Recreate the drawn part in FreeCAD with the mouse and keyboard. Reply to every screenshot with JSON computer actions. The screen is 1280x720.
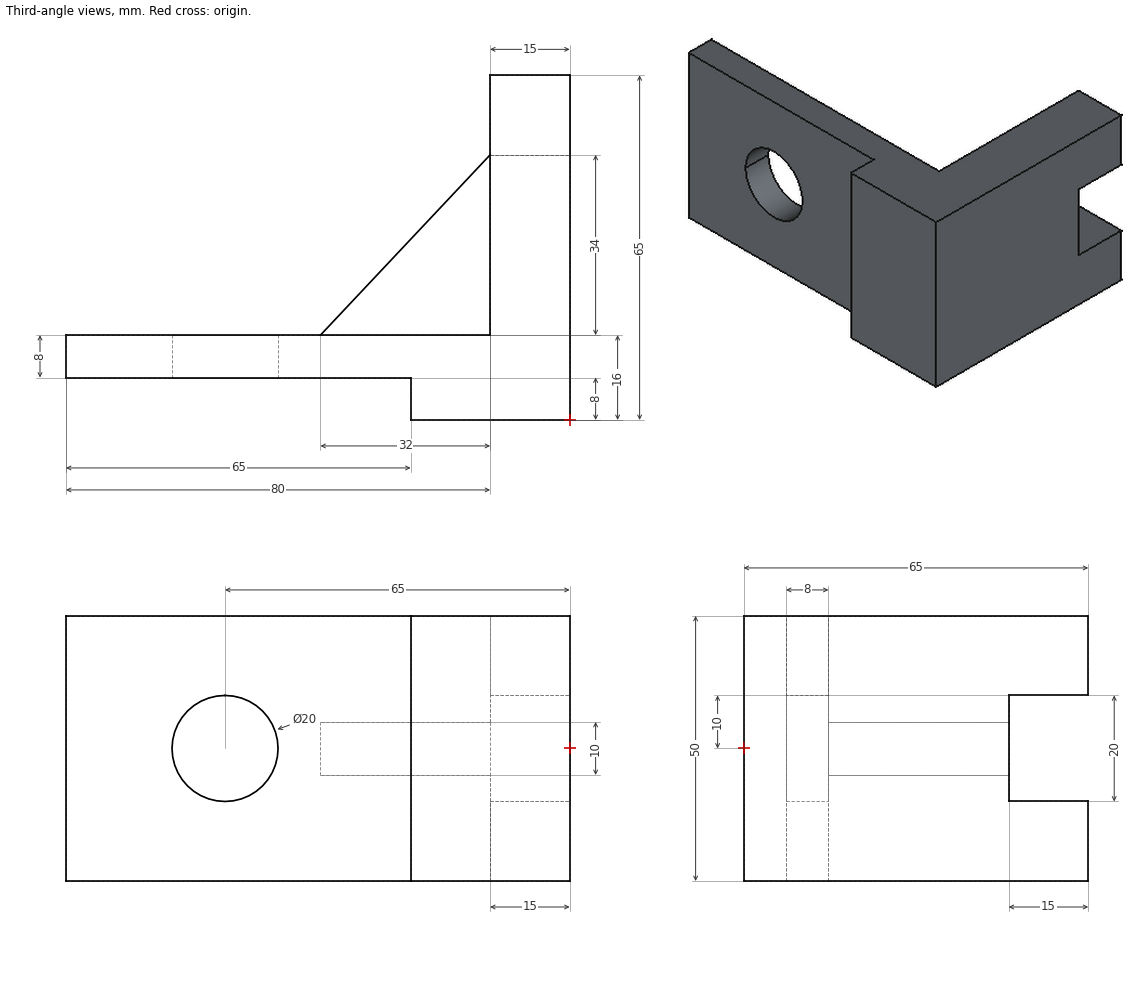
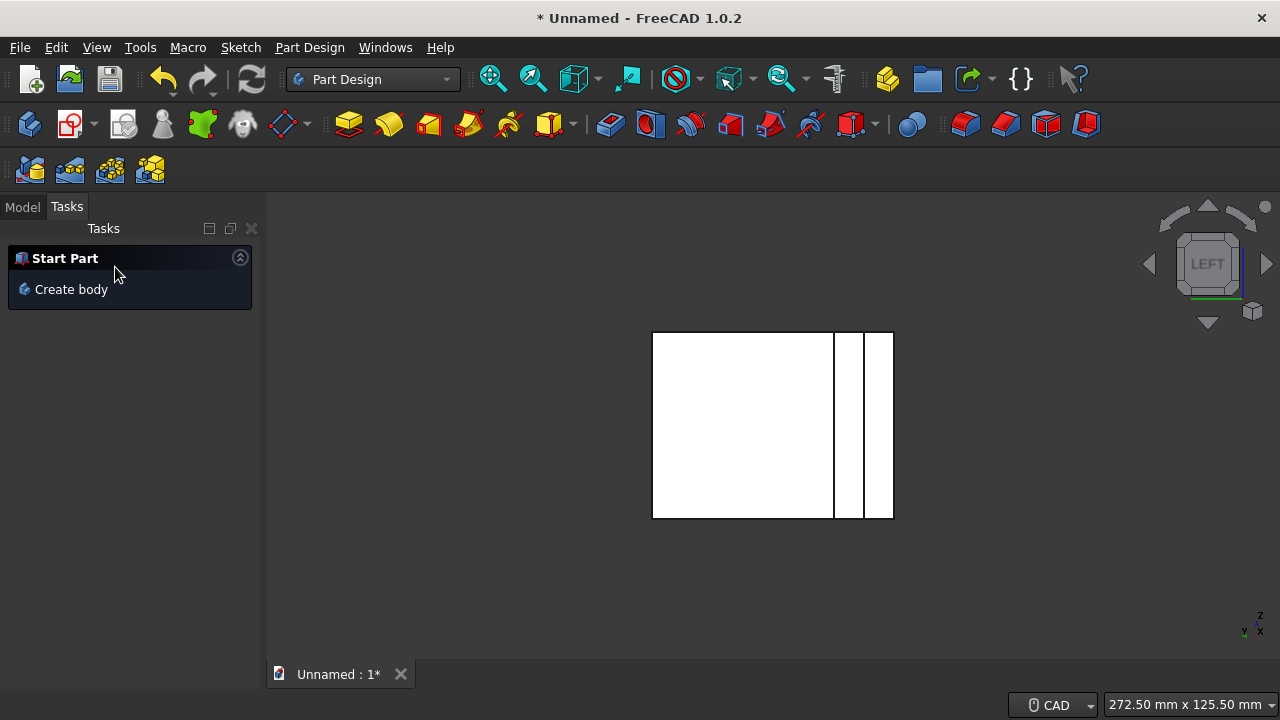
{"action": "left_click", "coordinate": [743, 424]}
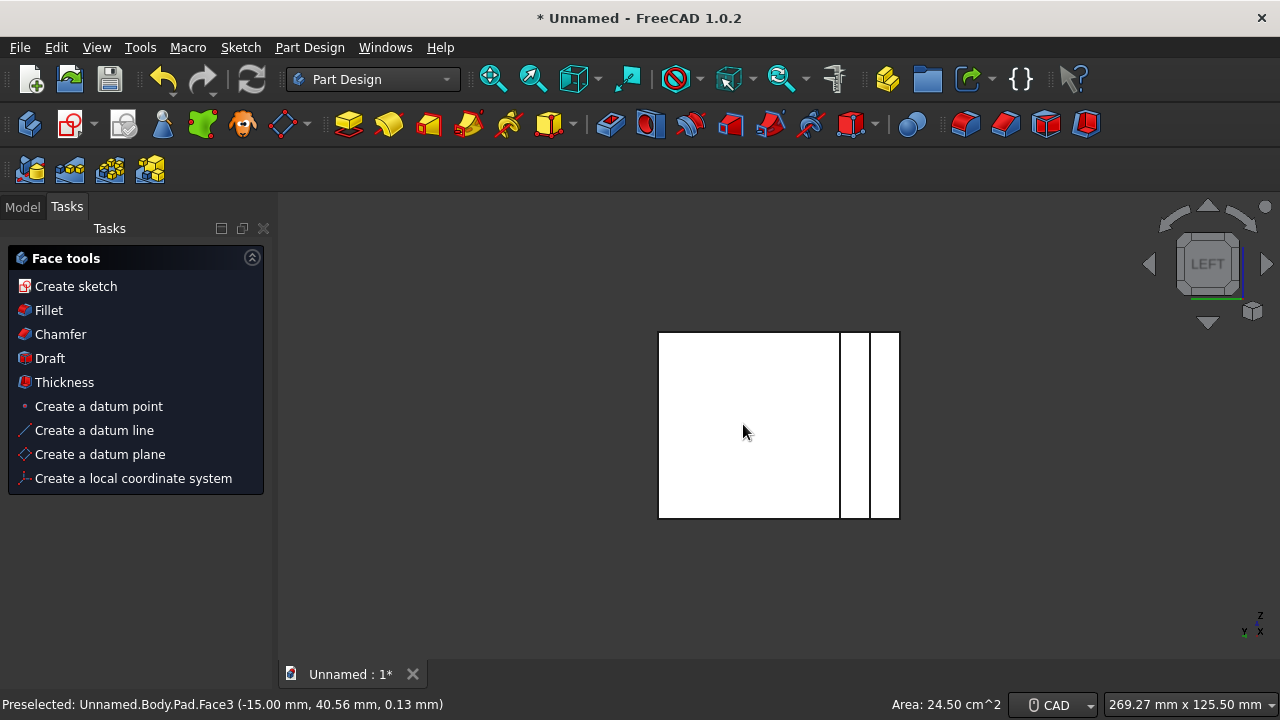
{"action": "left_click", "coordinate": [70, 124]}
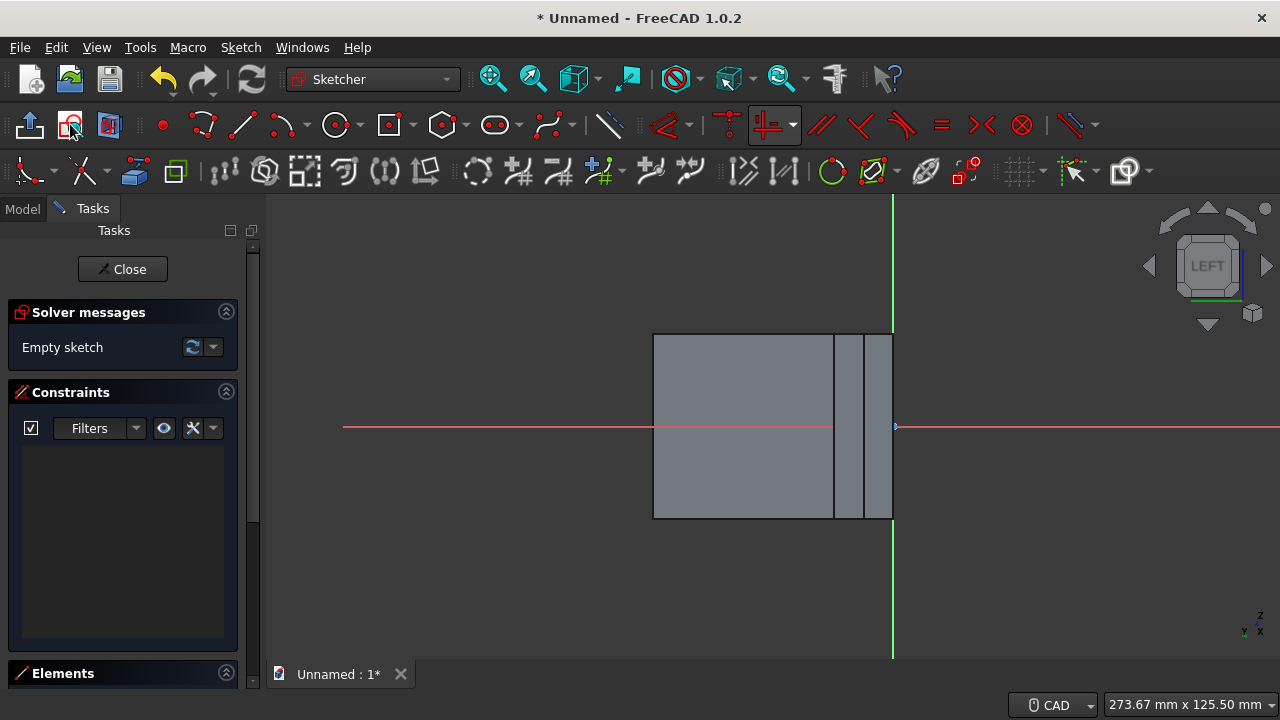
{"action": "scroll", "coordinate": [672, 426], "scroll_direction": "up", "scroll_amount": 7}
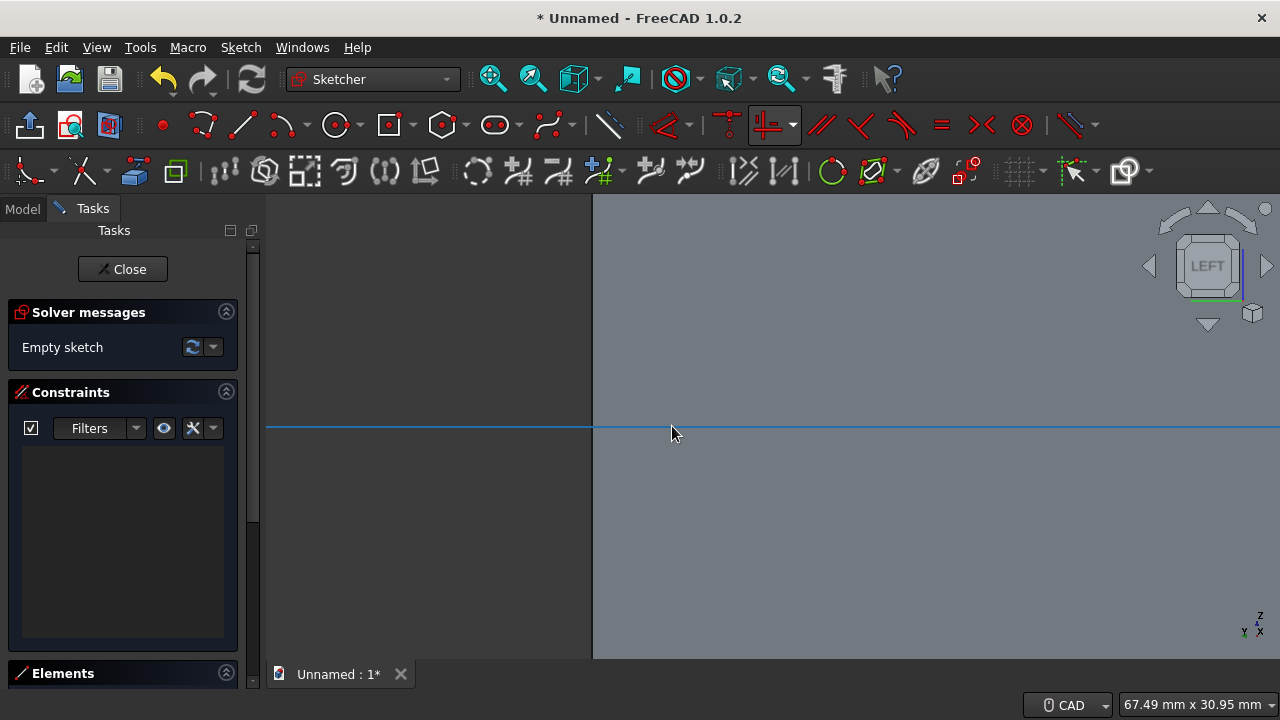
{"action": "left_click", "coordinate": [416, 126]}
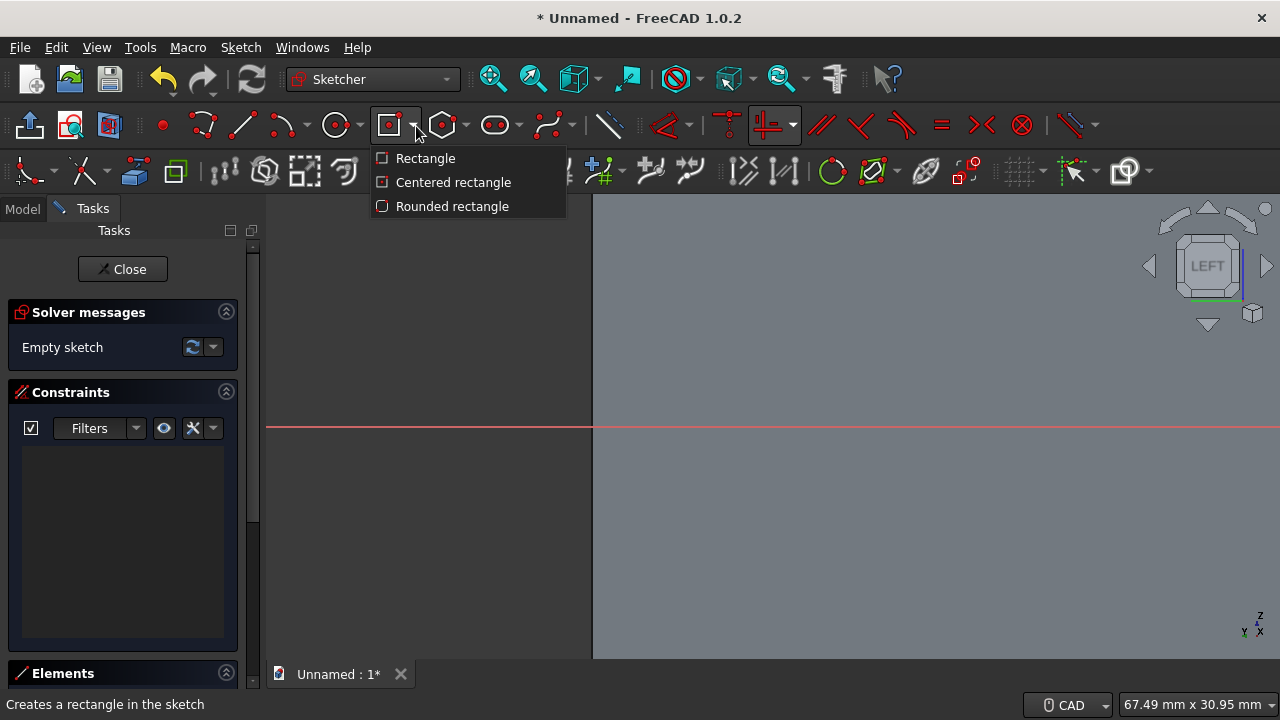
{"action": "left_click", "coordinate": [468, 158]}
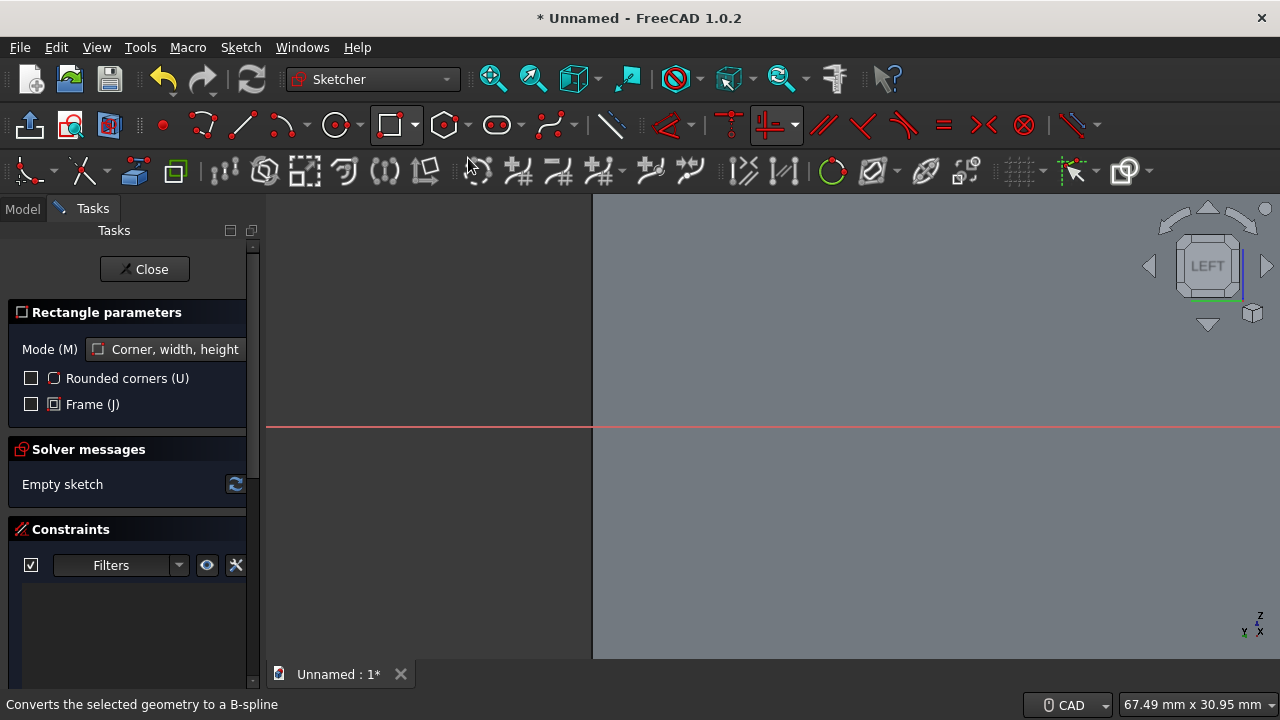
{"action": "left_click", "coordinate": [592, 276]}
{"action": "mouse_move", "coordinate": [817, 577]}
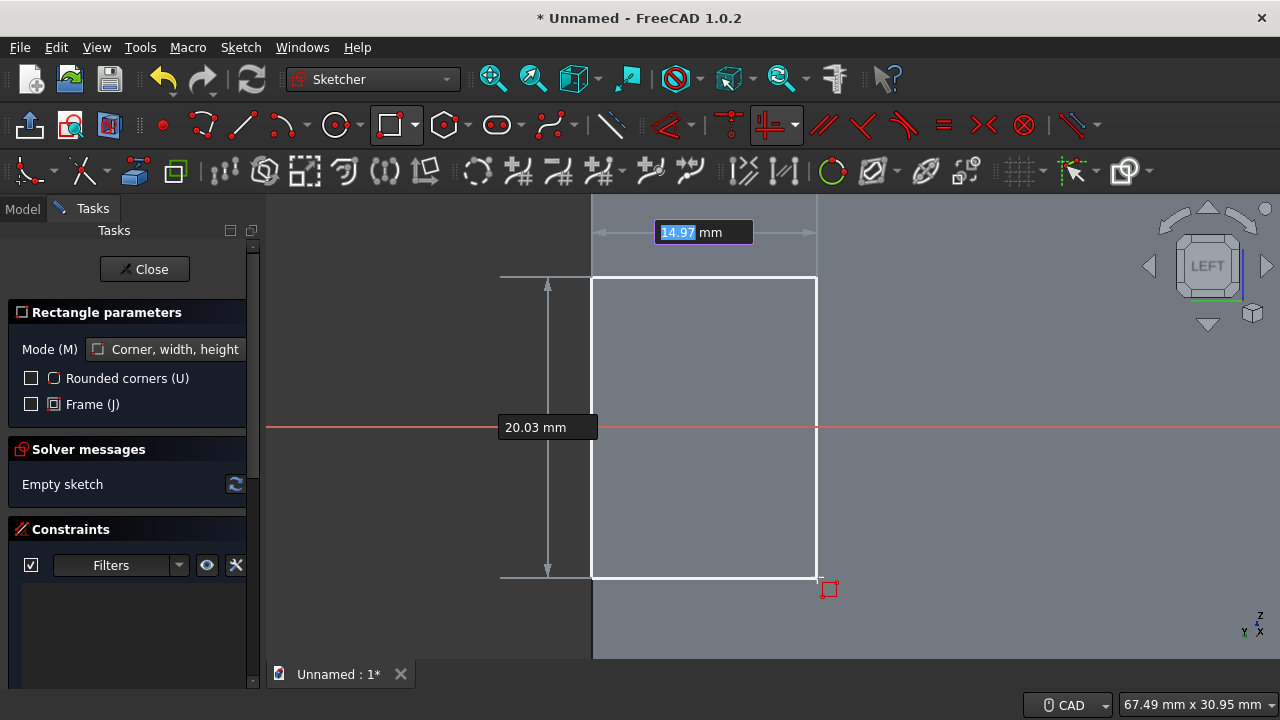
{"action": "type", "text": "15"}
{"action": "key", "text": "Tab"}
{"action": "type", "text": "20"}
{"action": "key", "text": "Return"}
{"action": "key", "text": "Escape"}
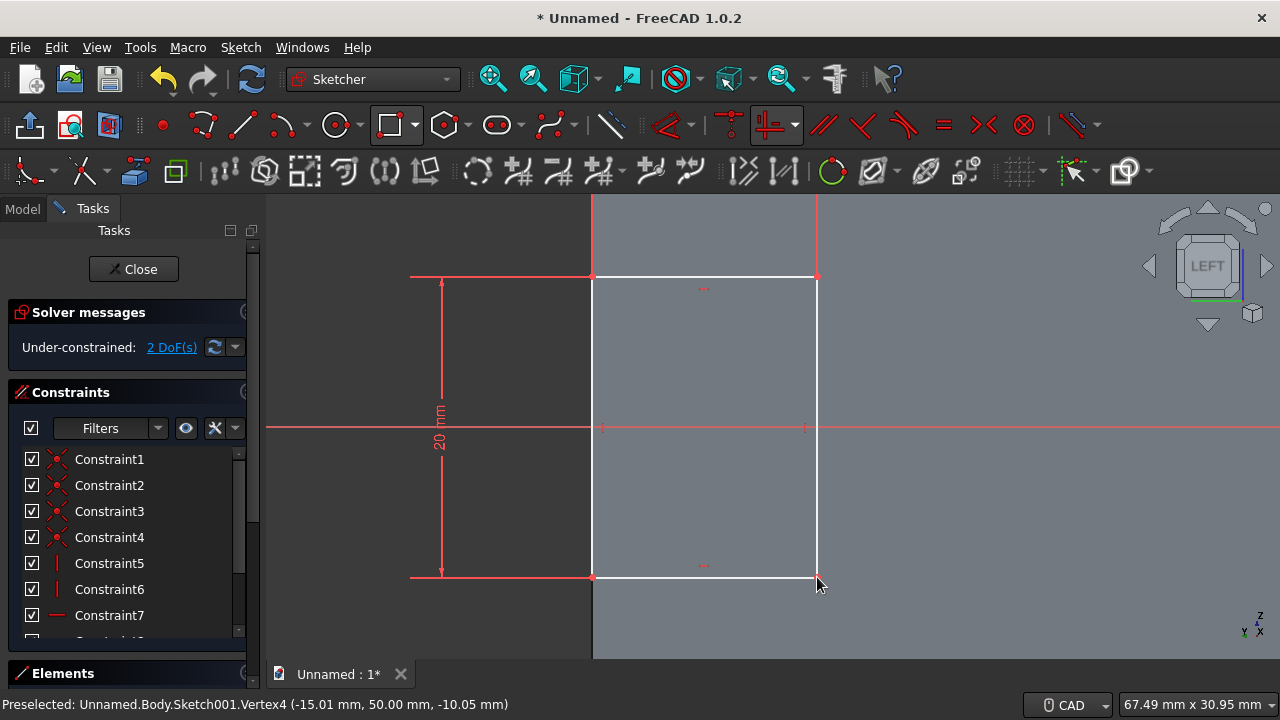
{"action": "key", "text": "d"}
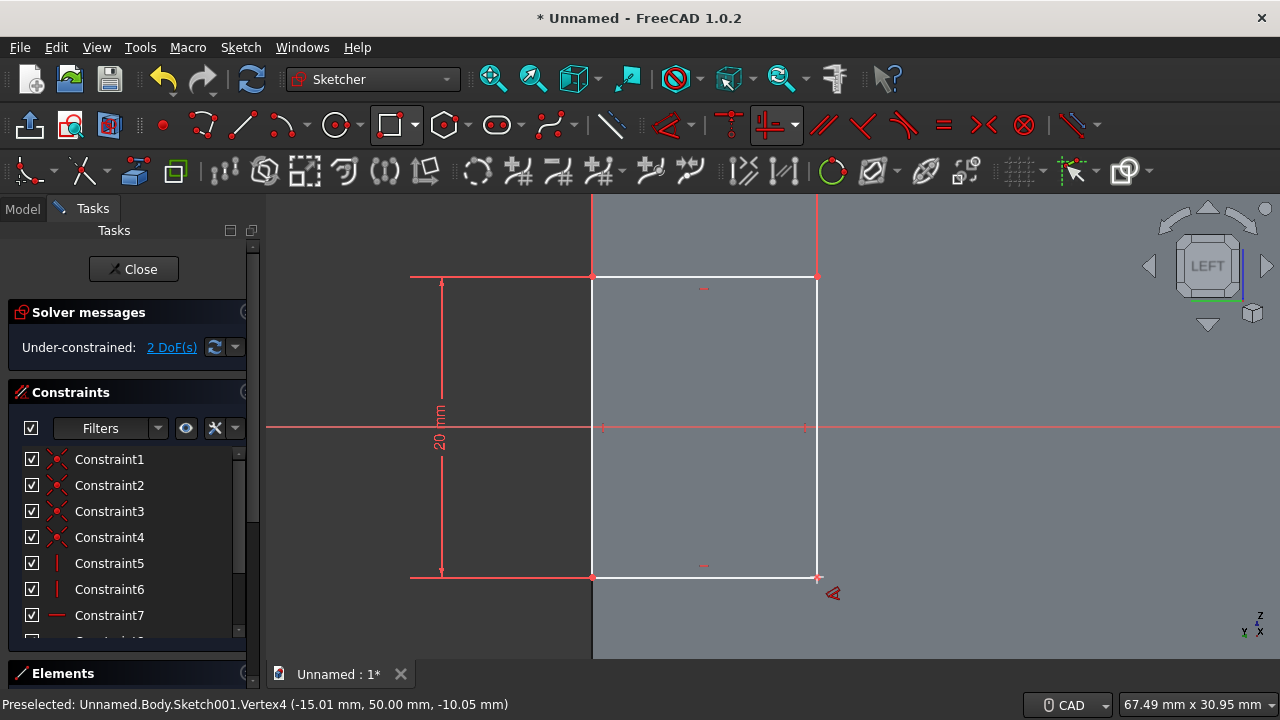
{"action": "left_click", "coordinate": [592, 277]}
{"action": "left_click", "coordinate": [853, 243]}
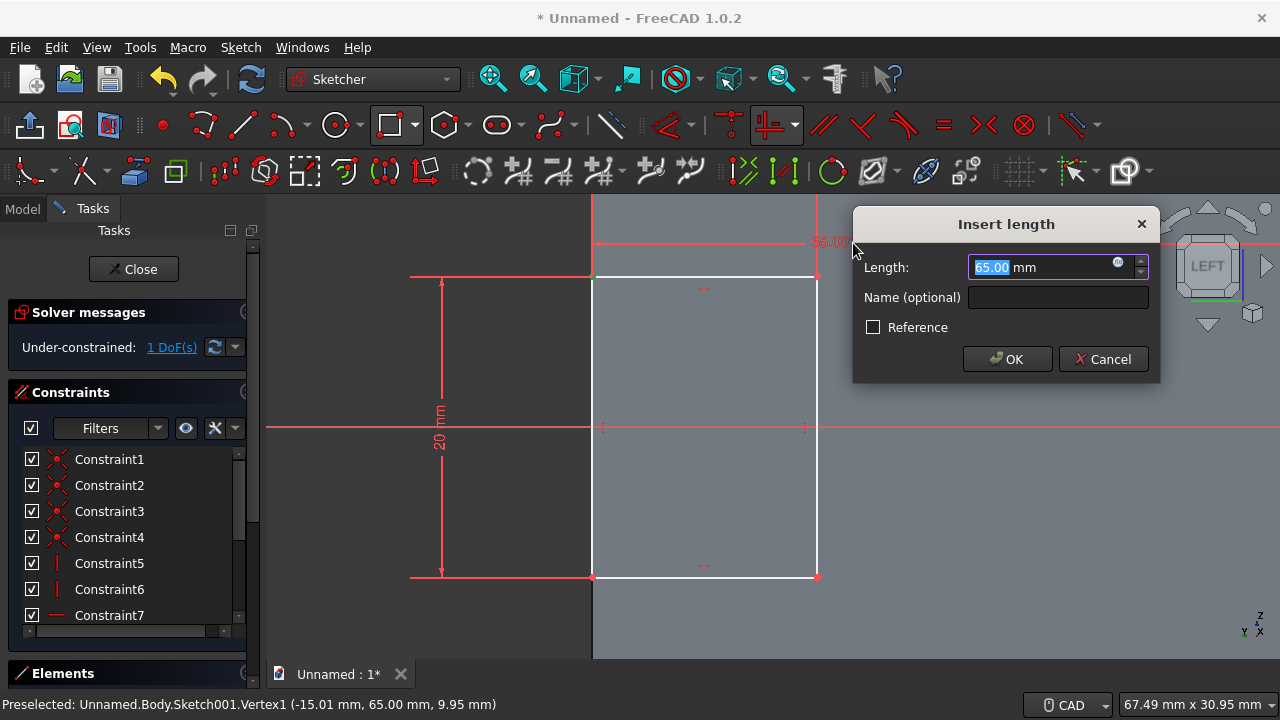
{"action": "type", "text": "65"}
{"action": "key", "text": "Return"}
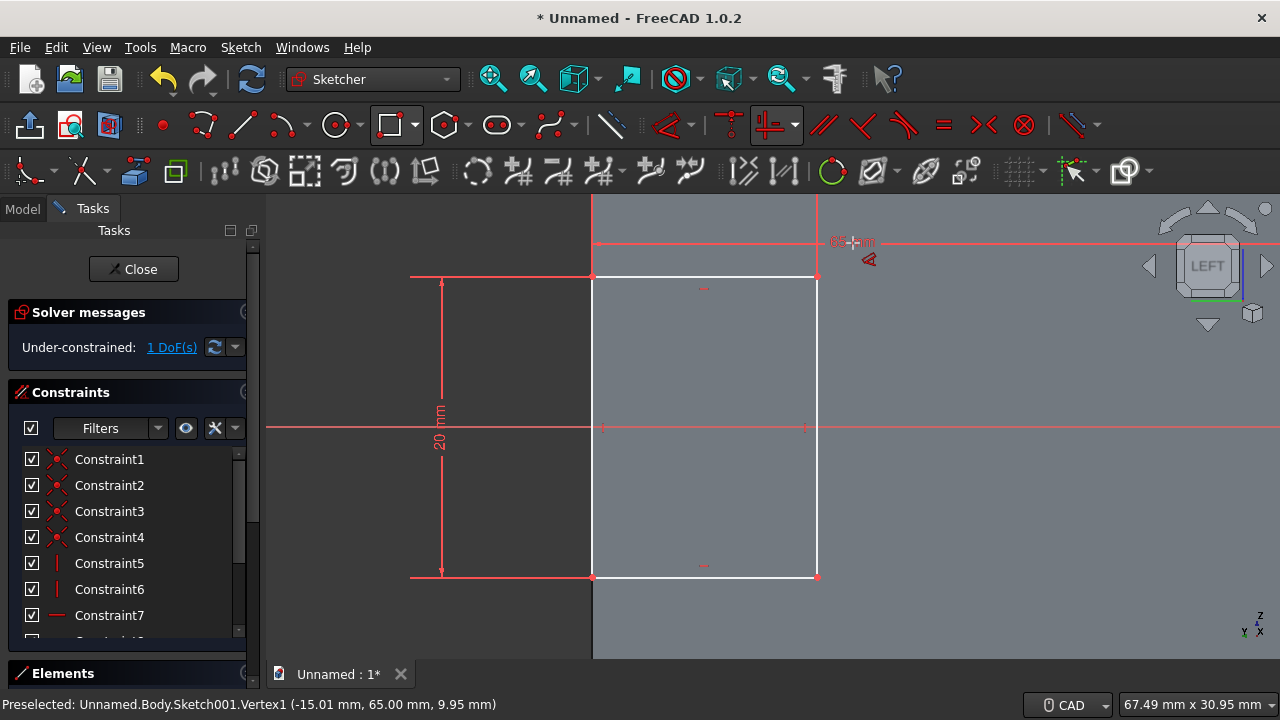
{"action": "left_click", "coordinate": [592, 277]}
{"action": "left_click", "coordinate": [558, 352]}